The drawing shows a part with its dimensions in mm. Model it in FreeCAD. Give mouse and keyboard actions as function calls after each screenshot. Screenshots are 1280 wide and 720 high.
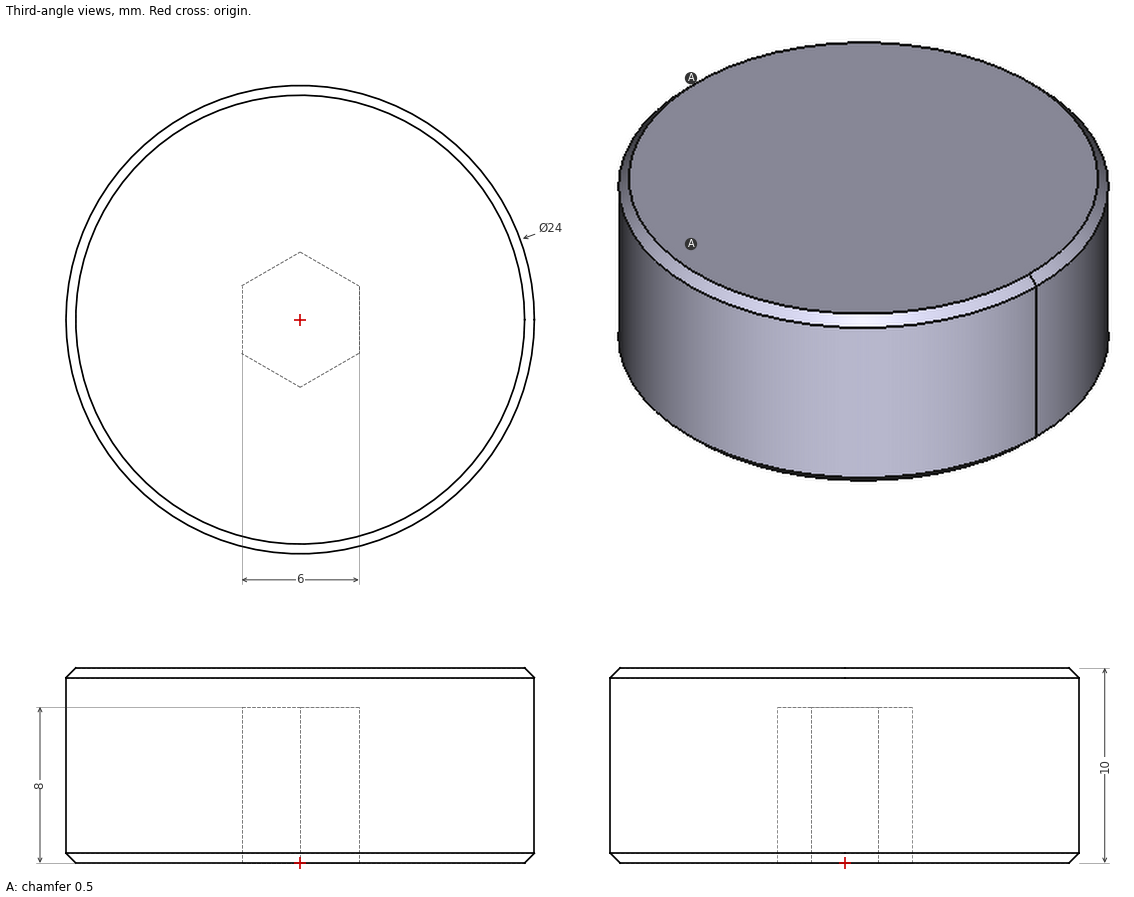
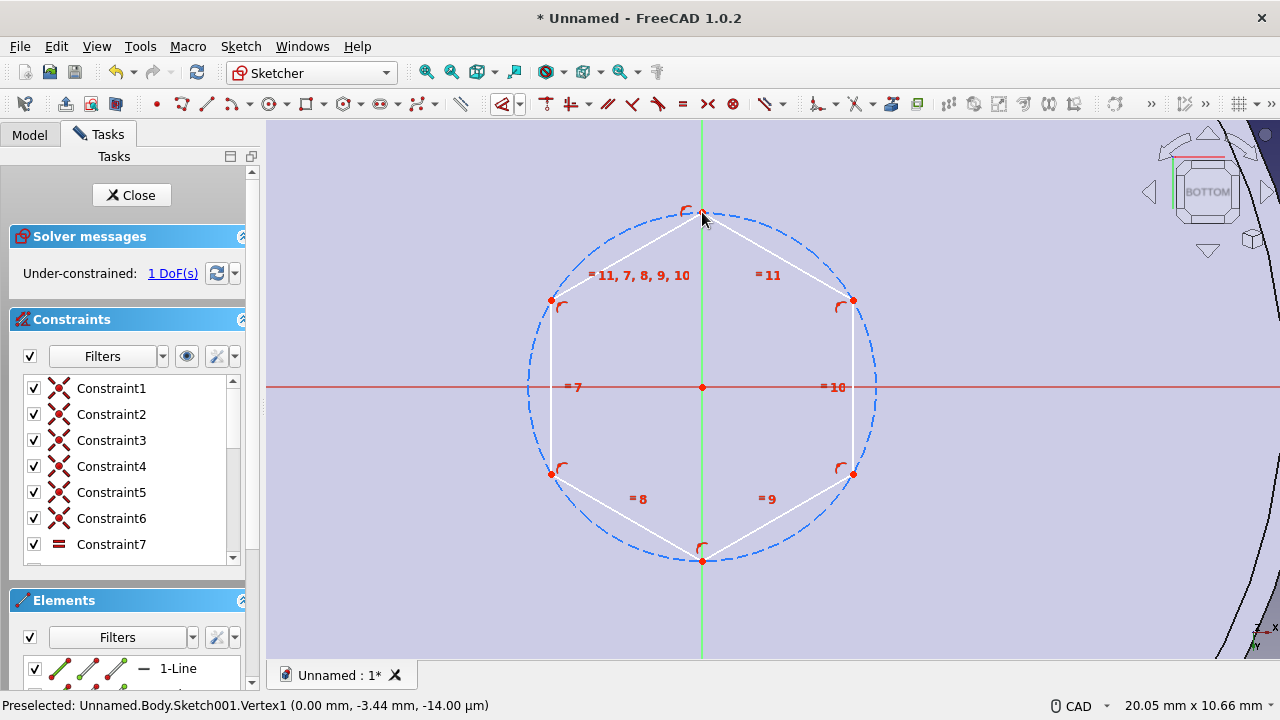
click(551, 300)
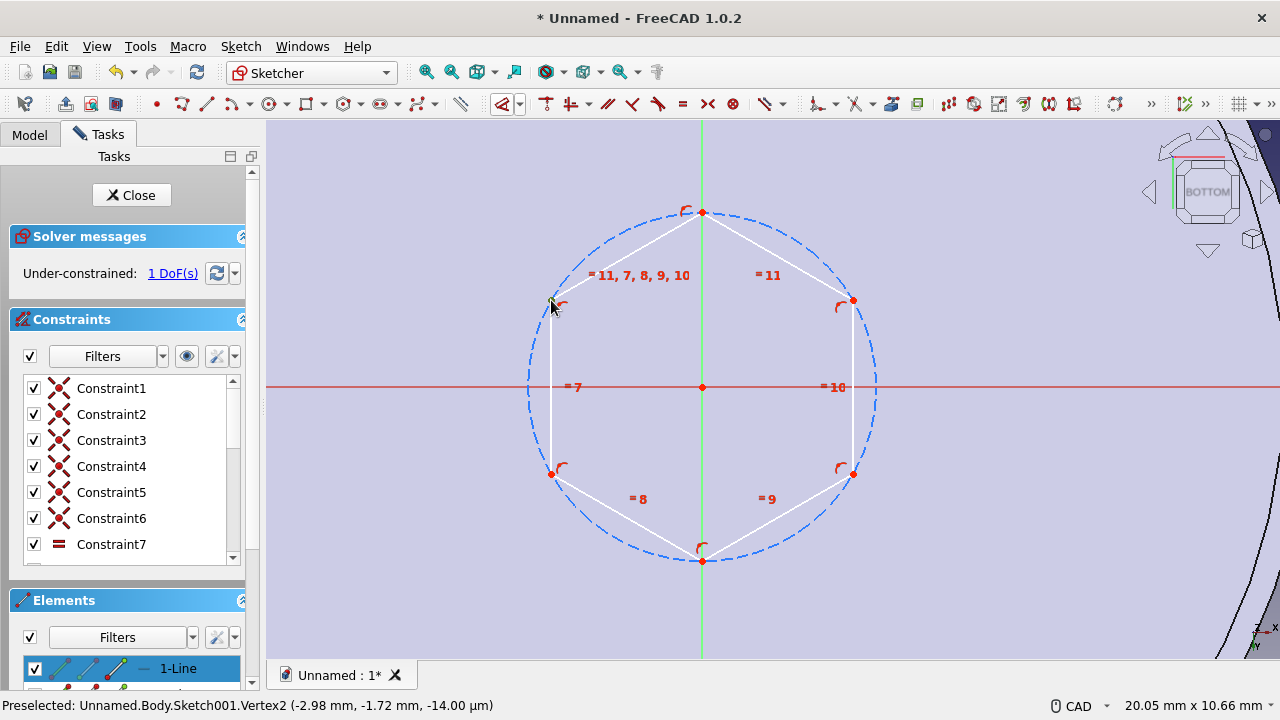
click(853, 474)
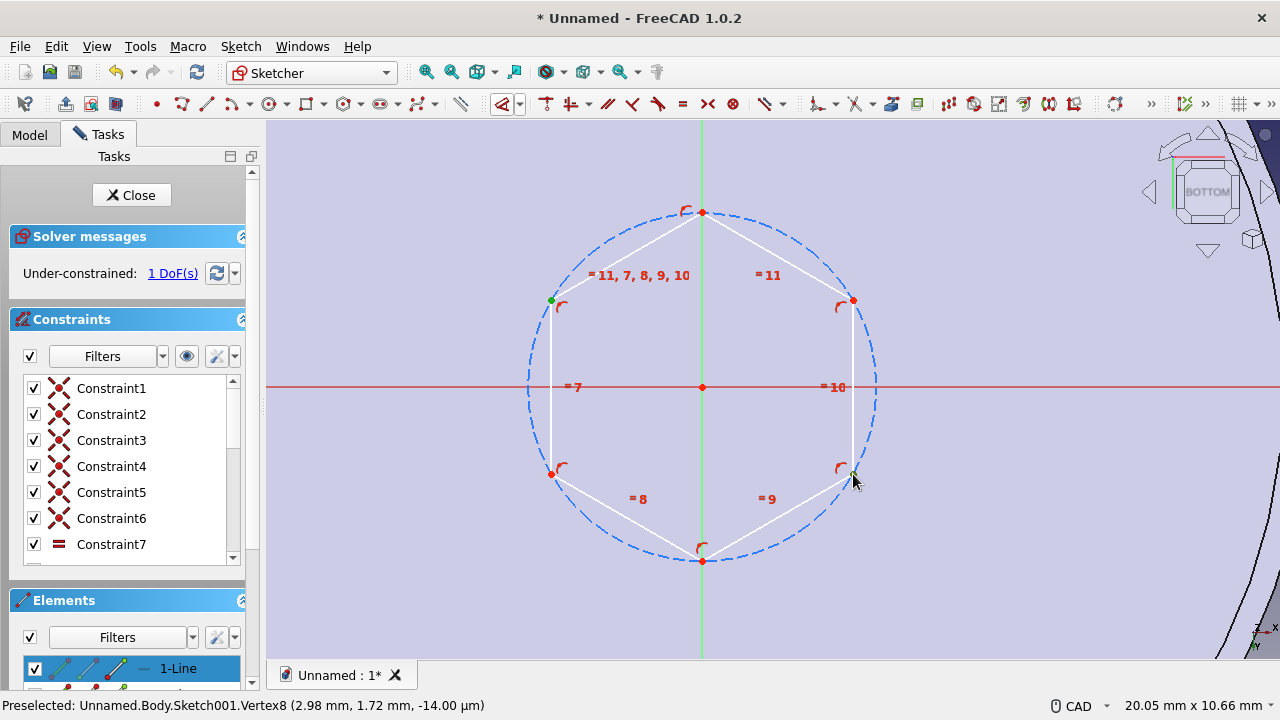
click(520, 104)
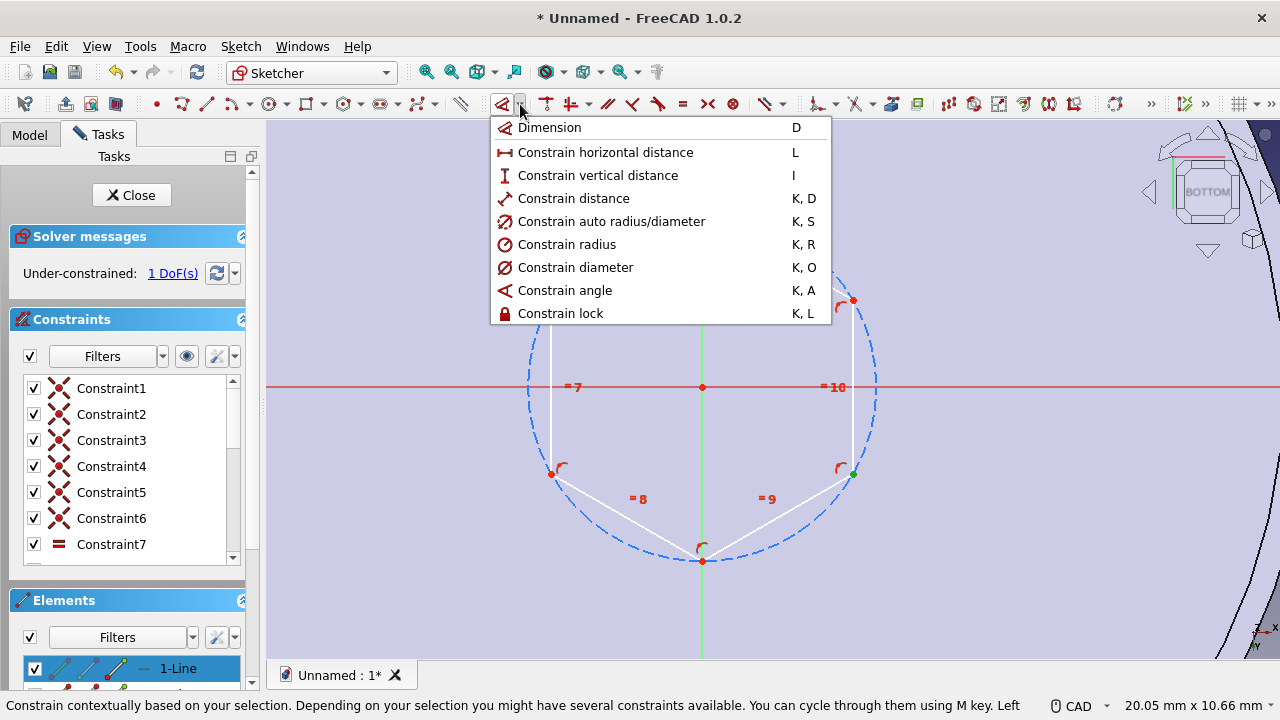
click(661, 152)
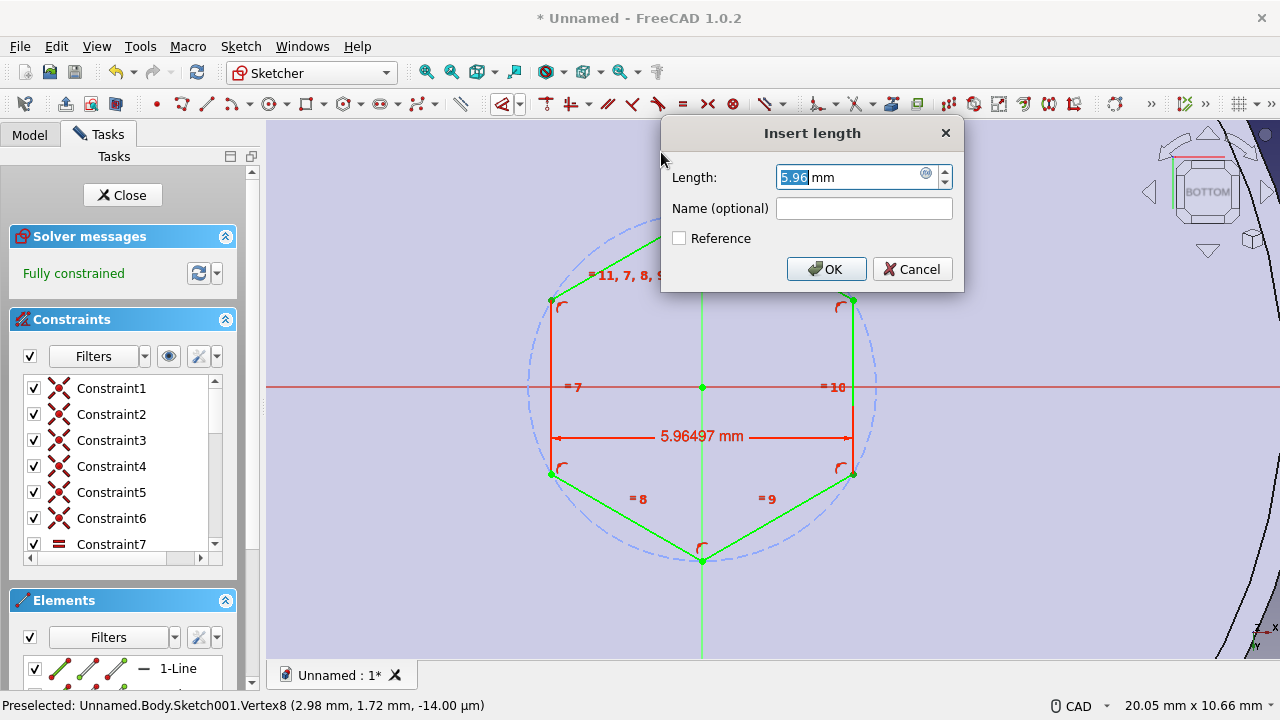
text(6)
key(Return)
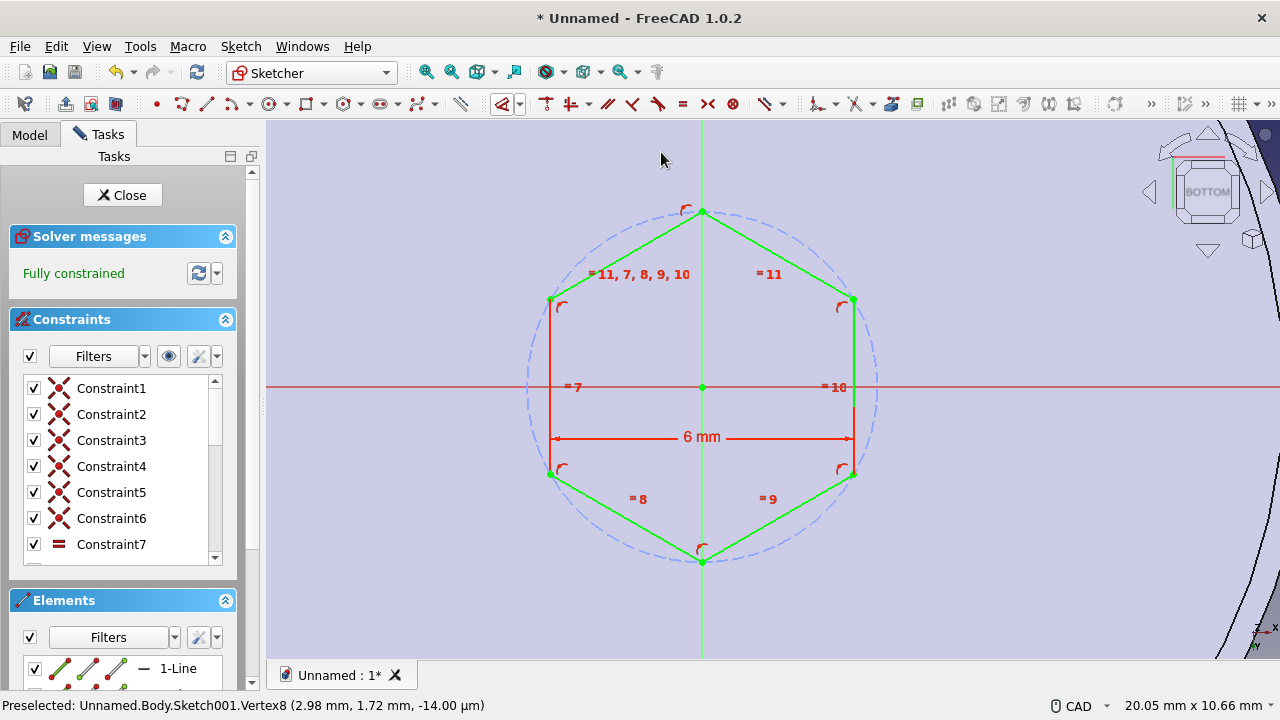
click(123, 195)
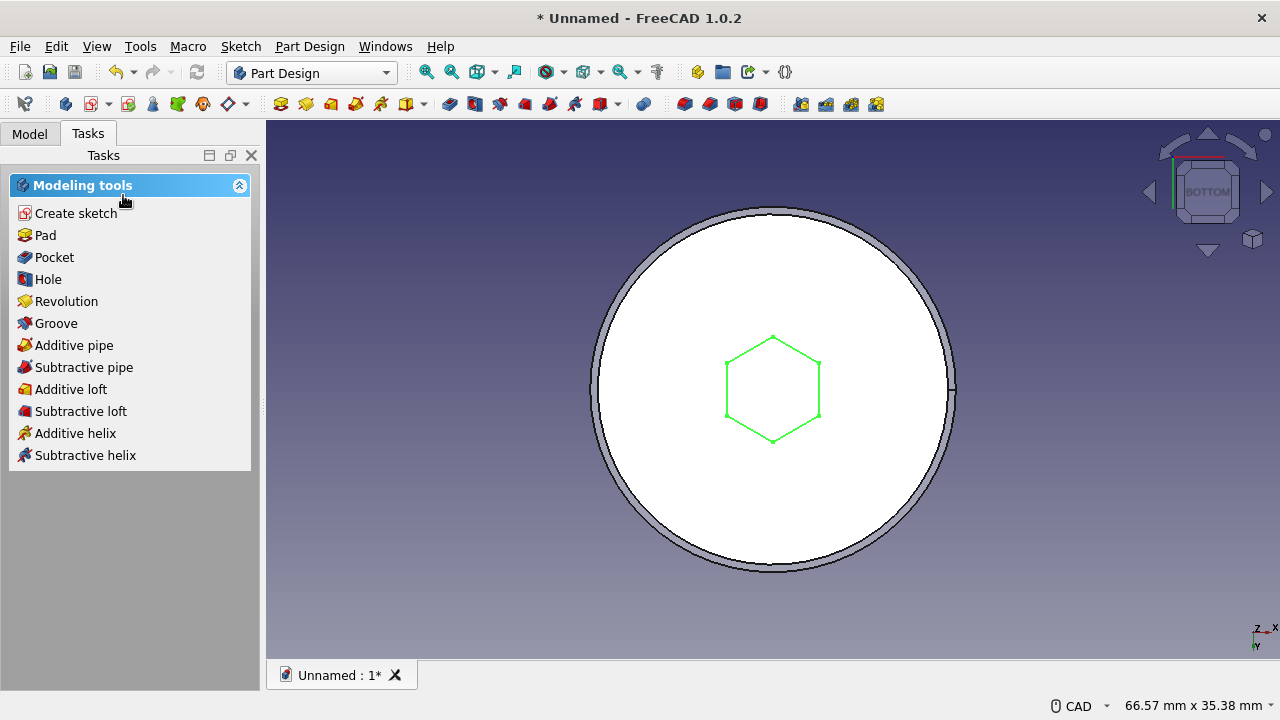
click(450, 104)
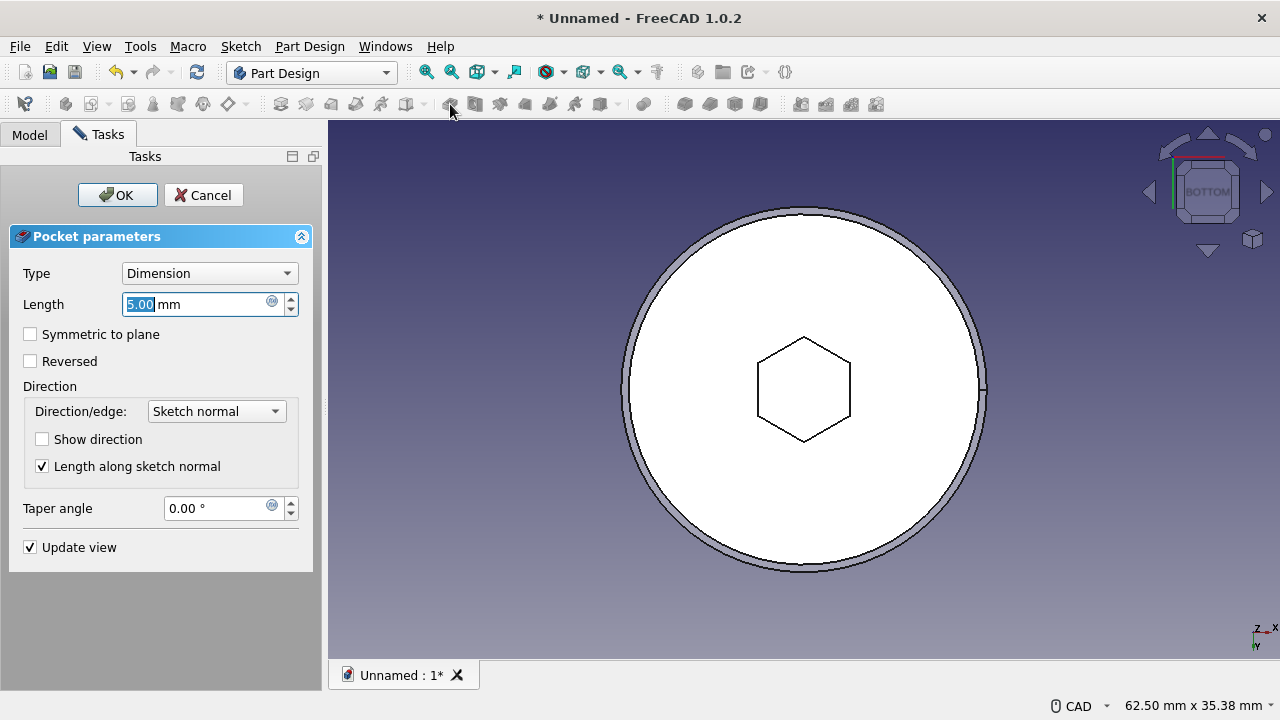
text(8)
key(Tab)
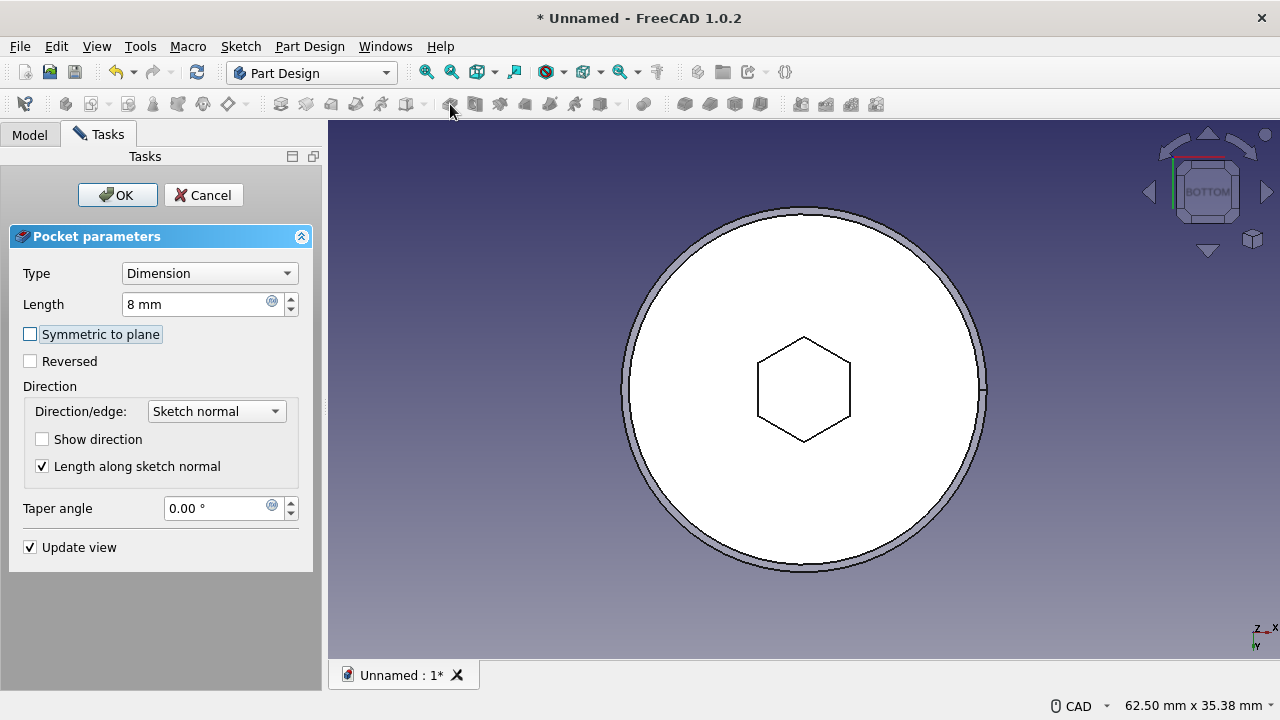
click(118, 195)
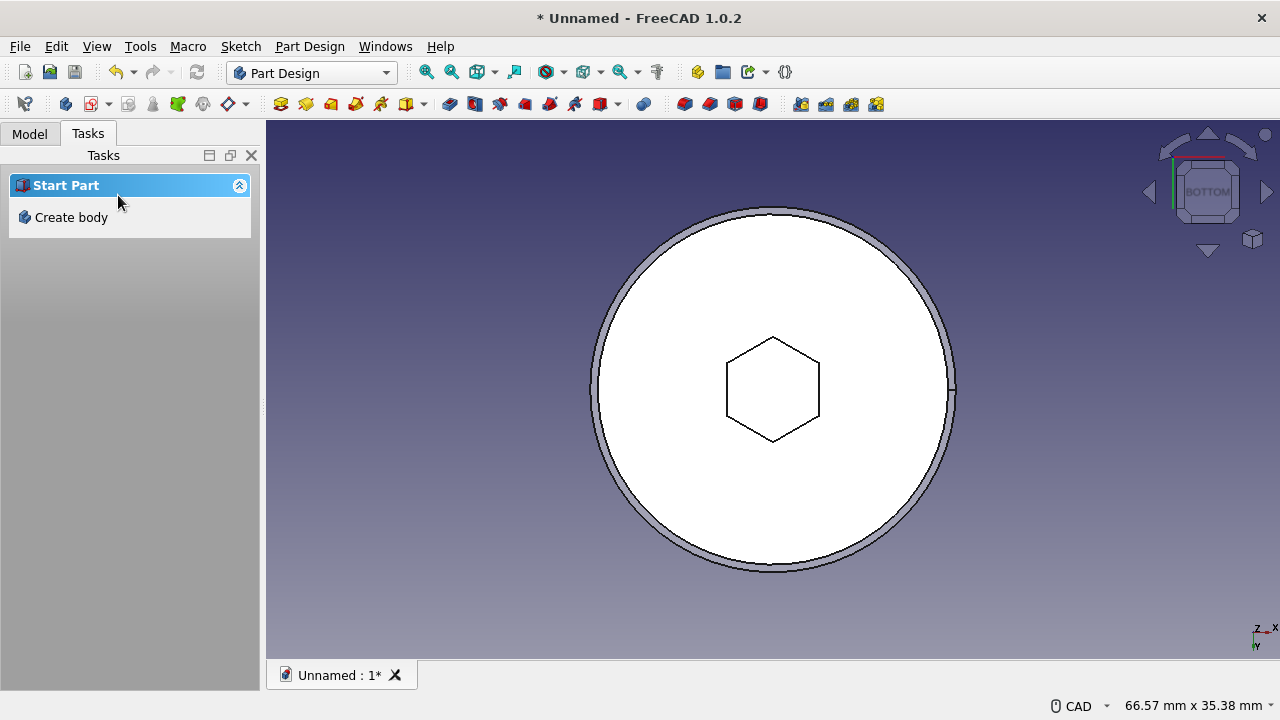
key(0)